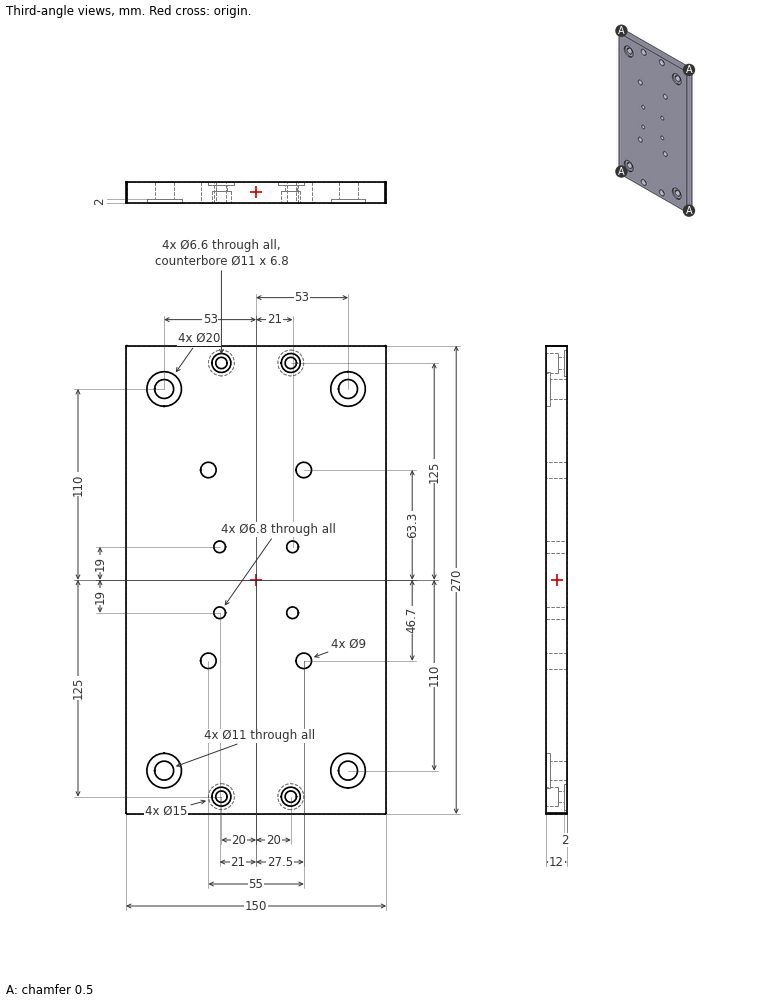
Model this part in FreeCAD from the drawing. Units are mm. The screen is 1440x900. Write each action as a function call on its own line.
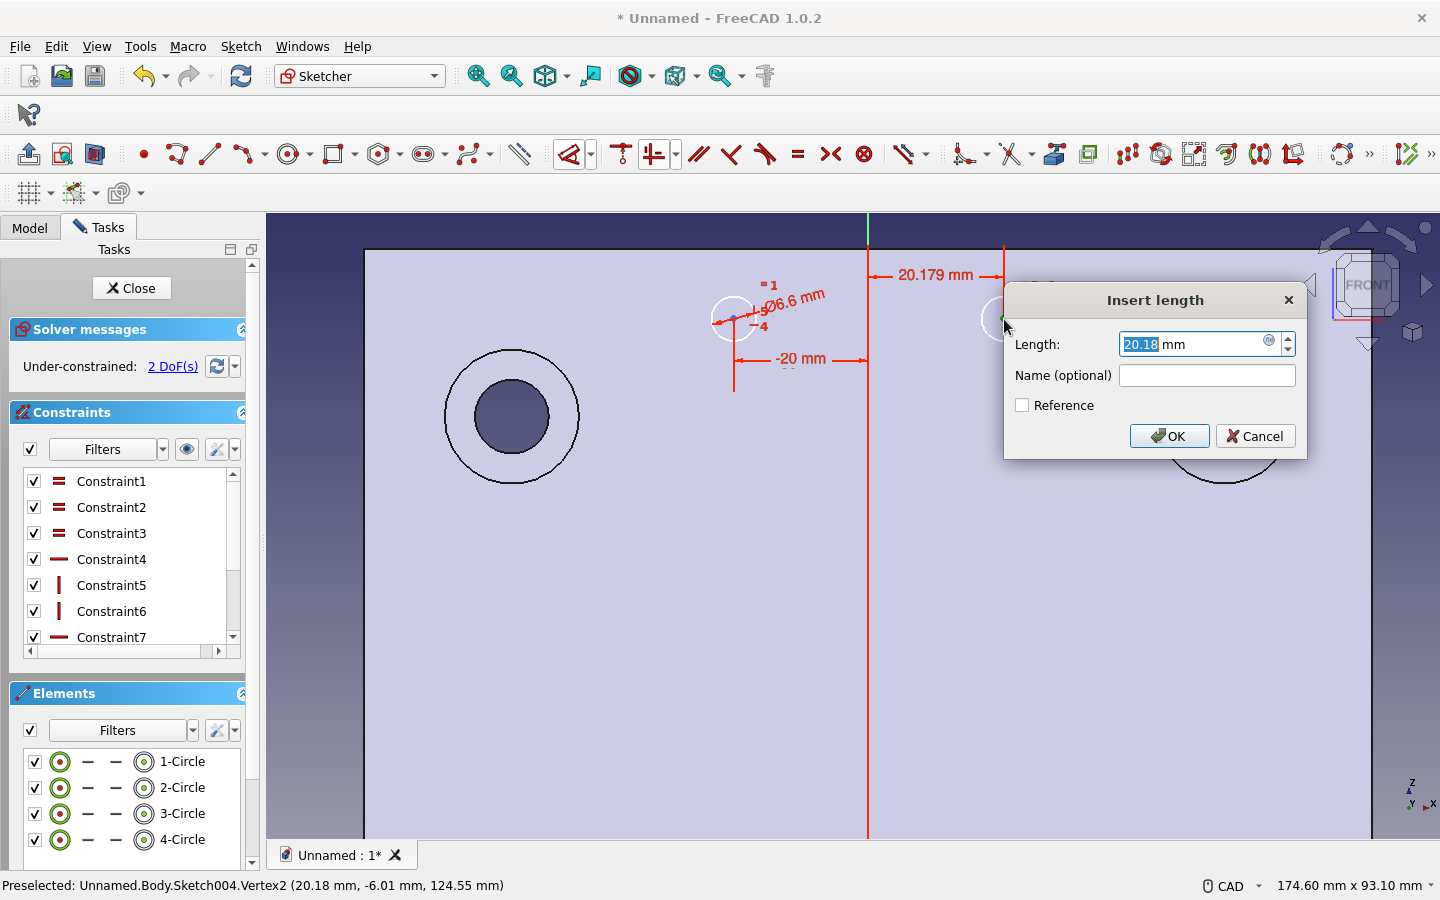
text(20)
key(Return)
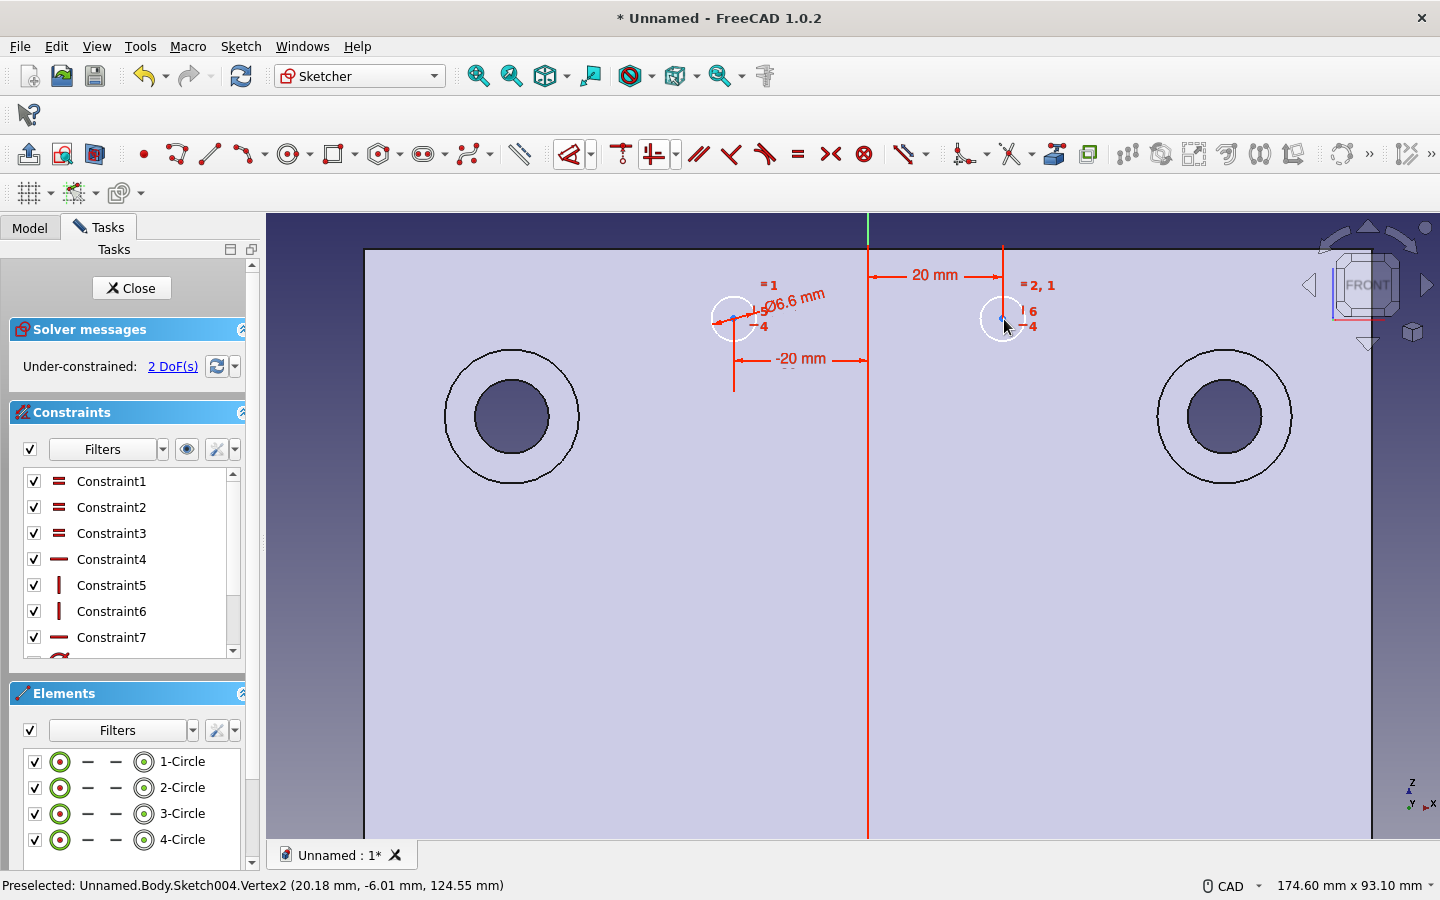
click(734, 319)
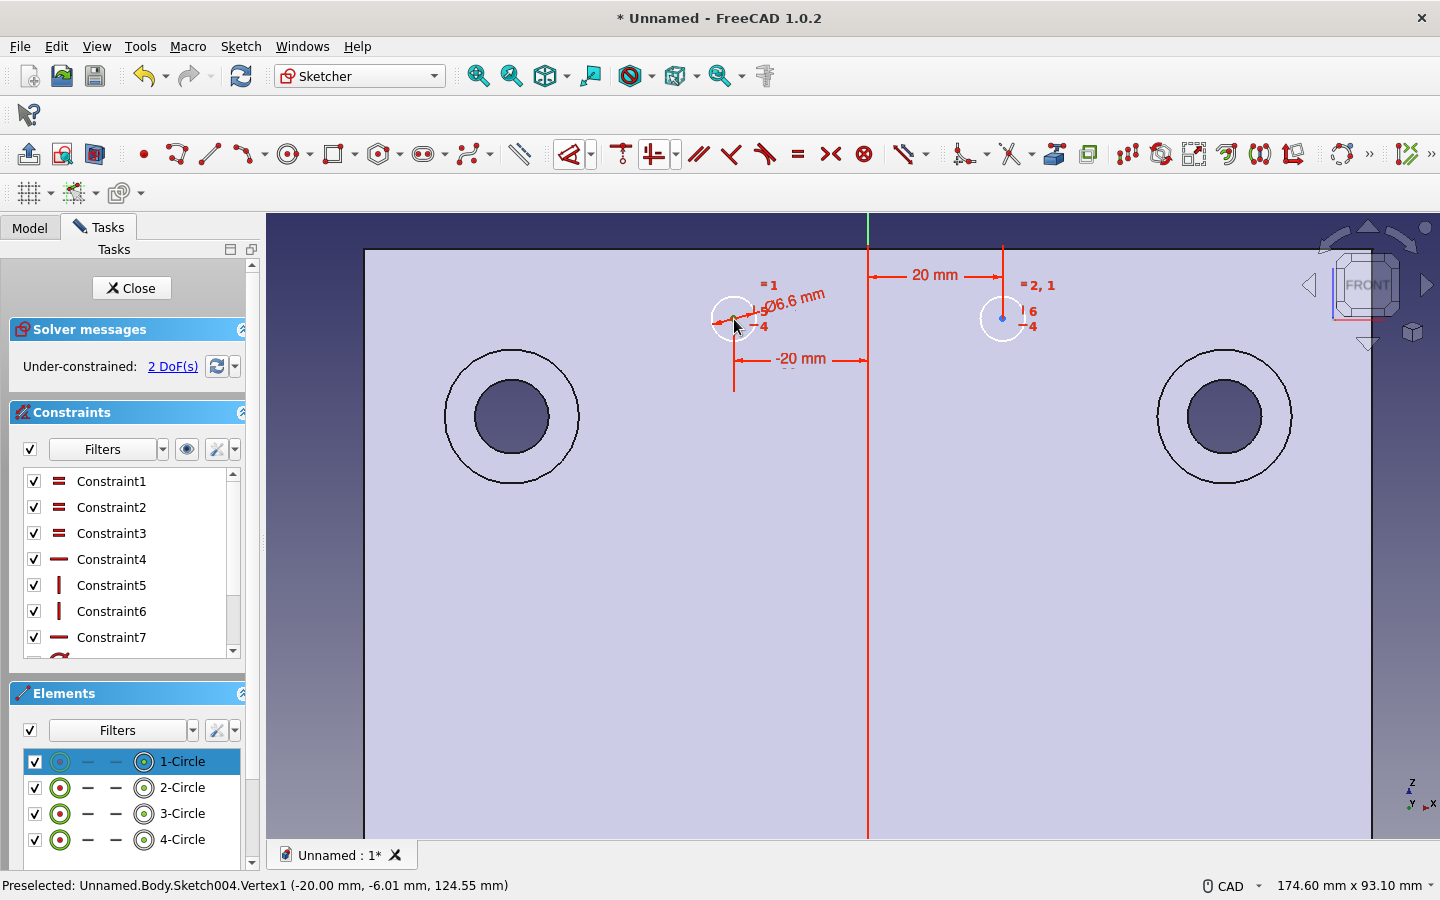
key(i)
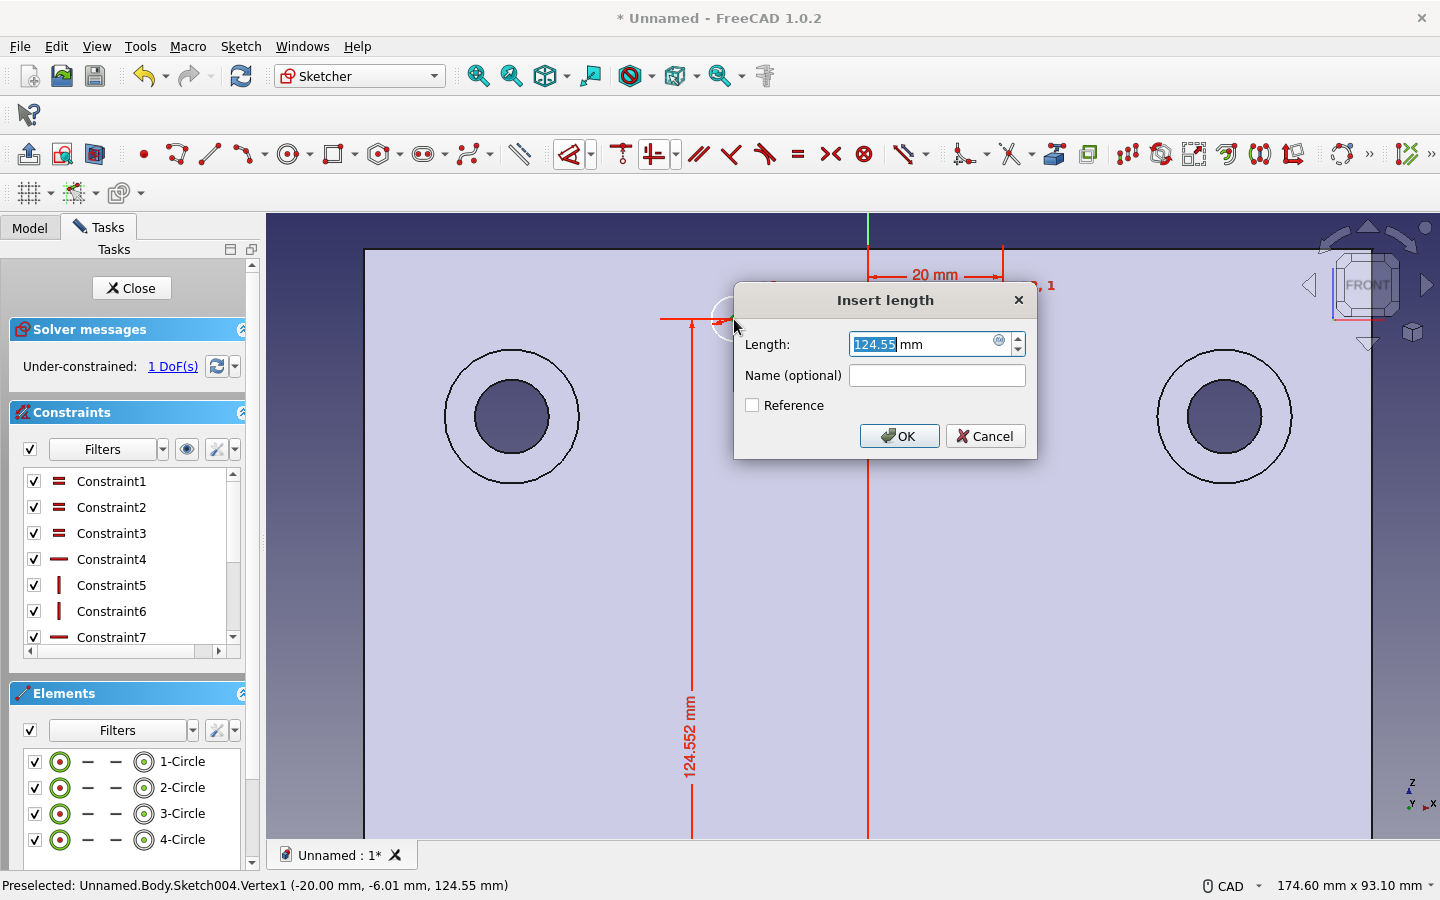
text(125)
key(Return)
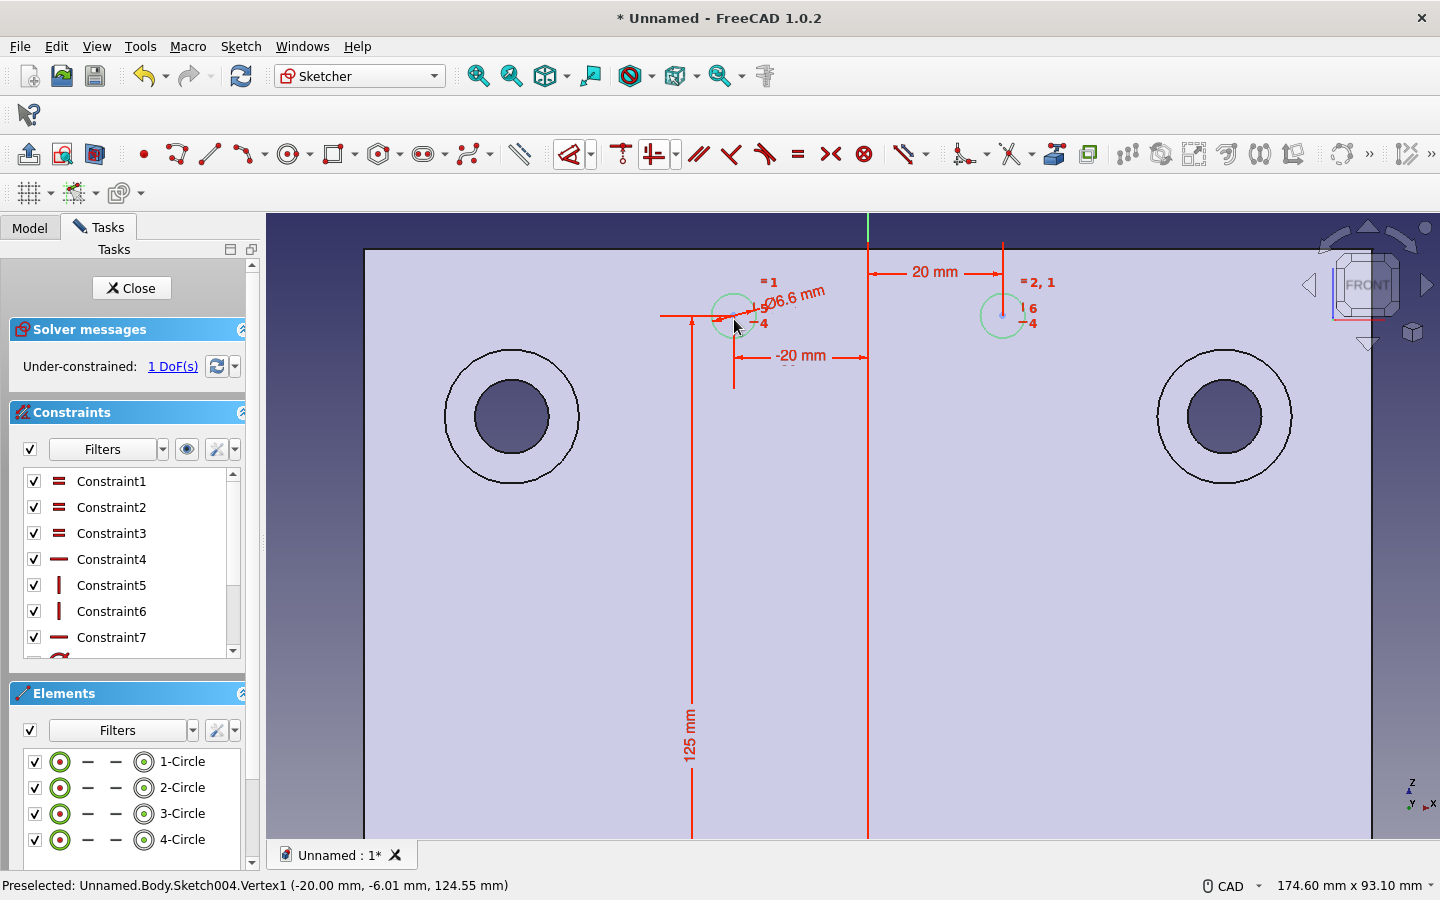
scroll(757, 320, down, 7)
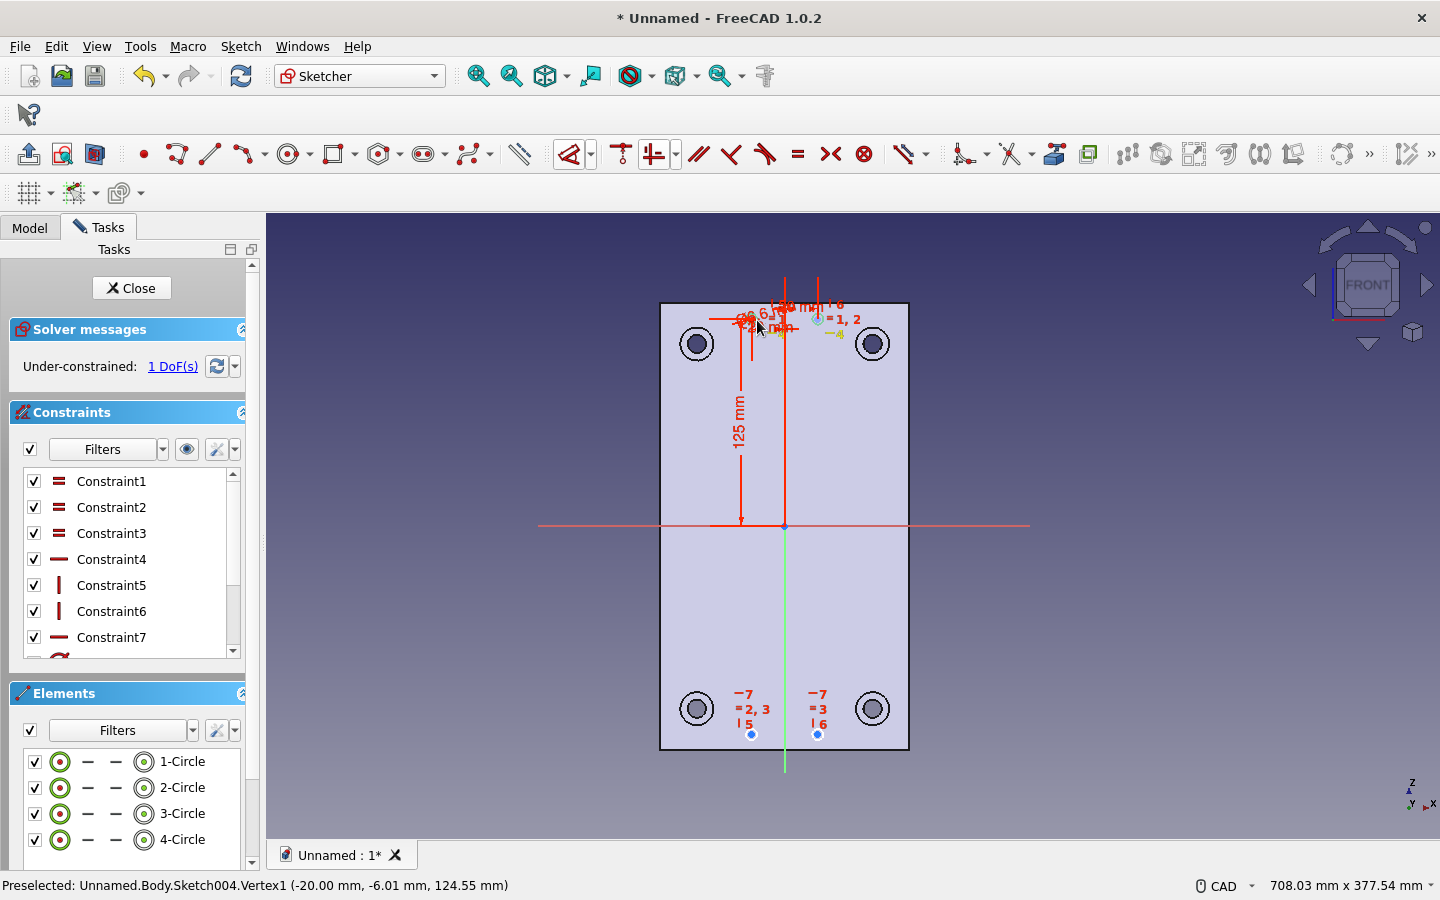
click(752, 735)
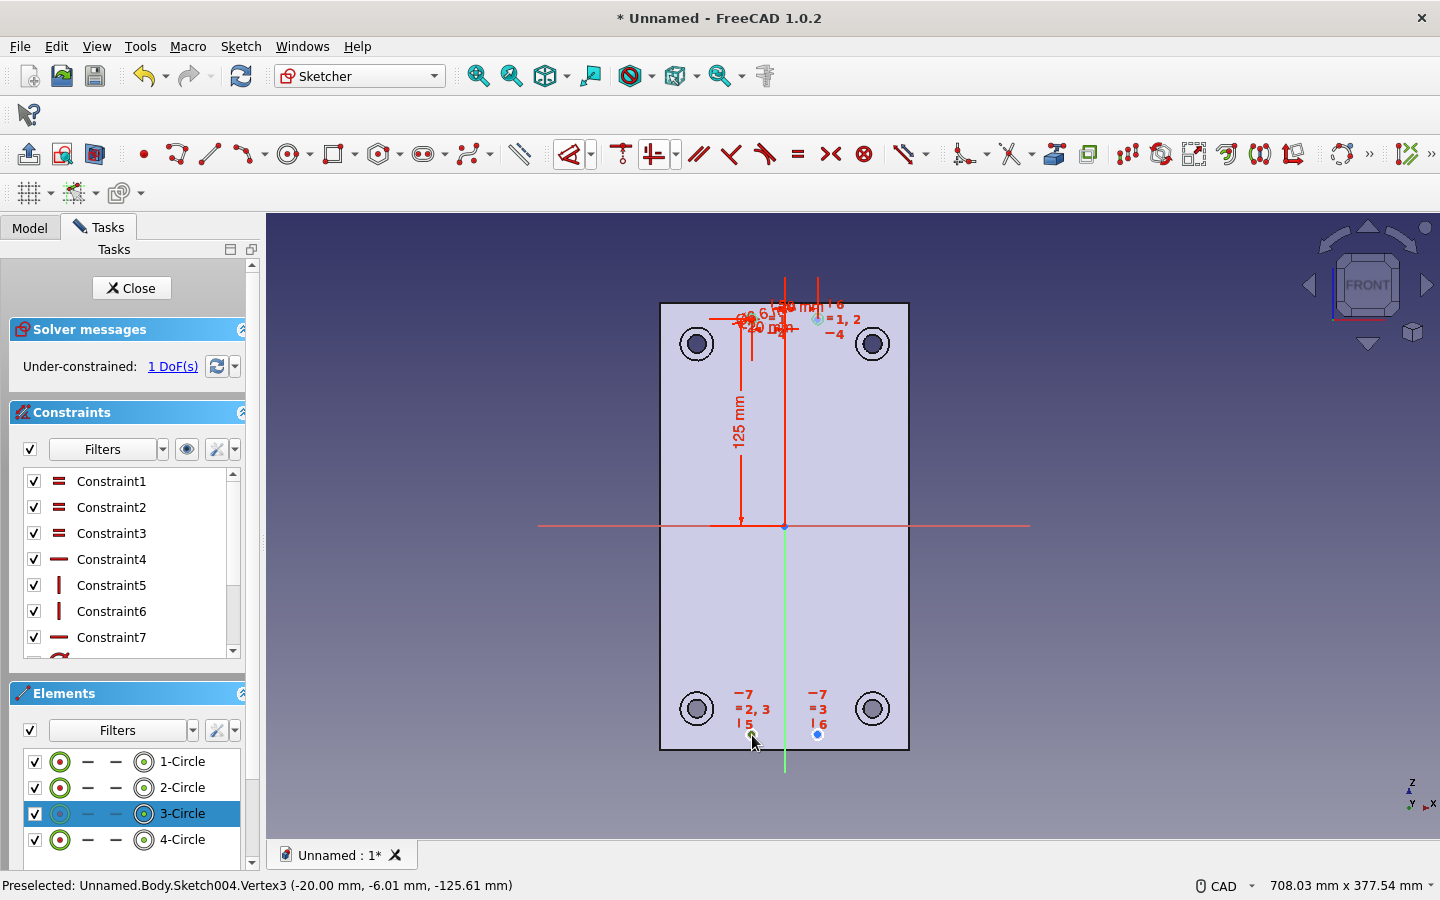
key(i)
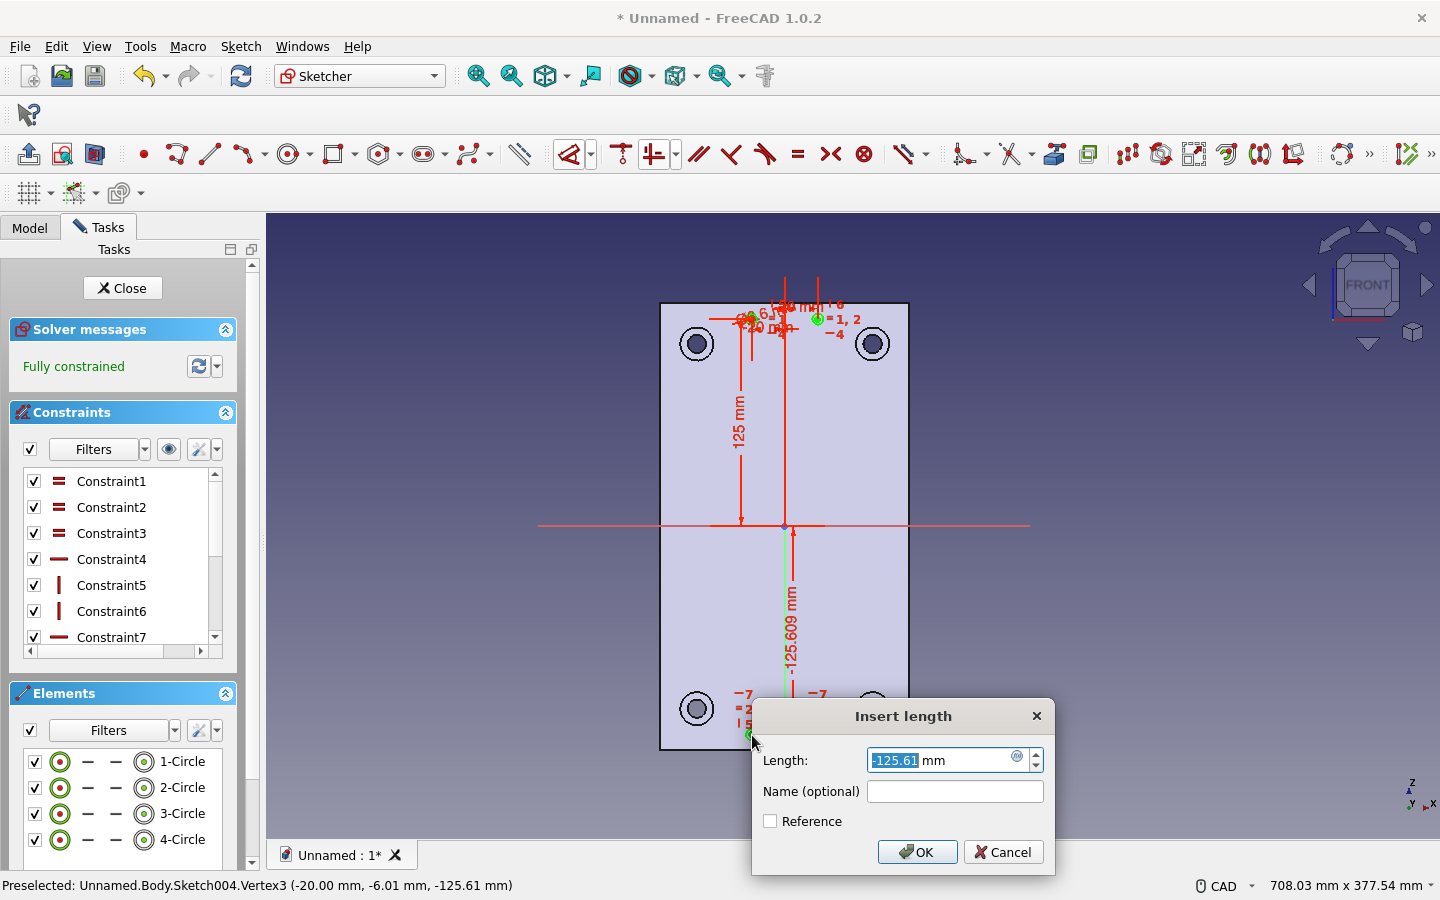
text(-125)
key(Return)